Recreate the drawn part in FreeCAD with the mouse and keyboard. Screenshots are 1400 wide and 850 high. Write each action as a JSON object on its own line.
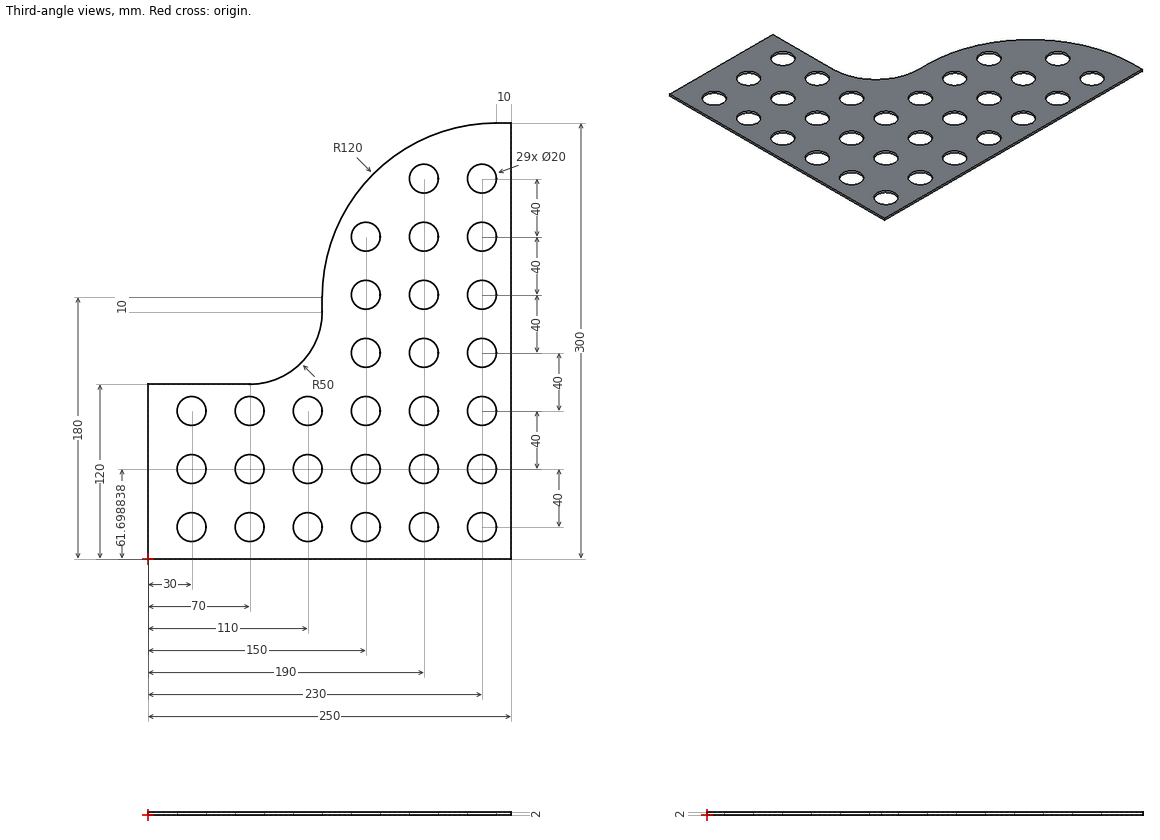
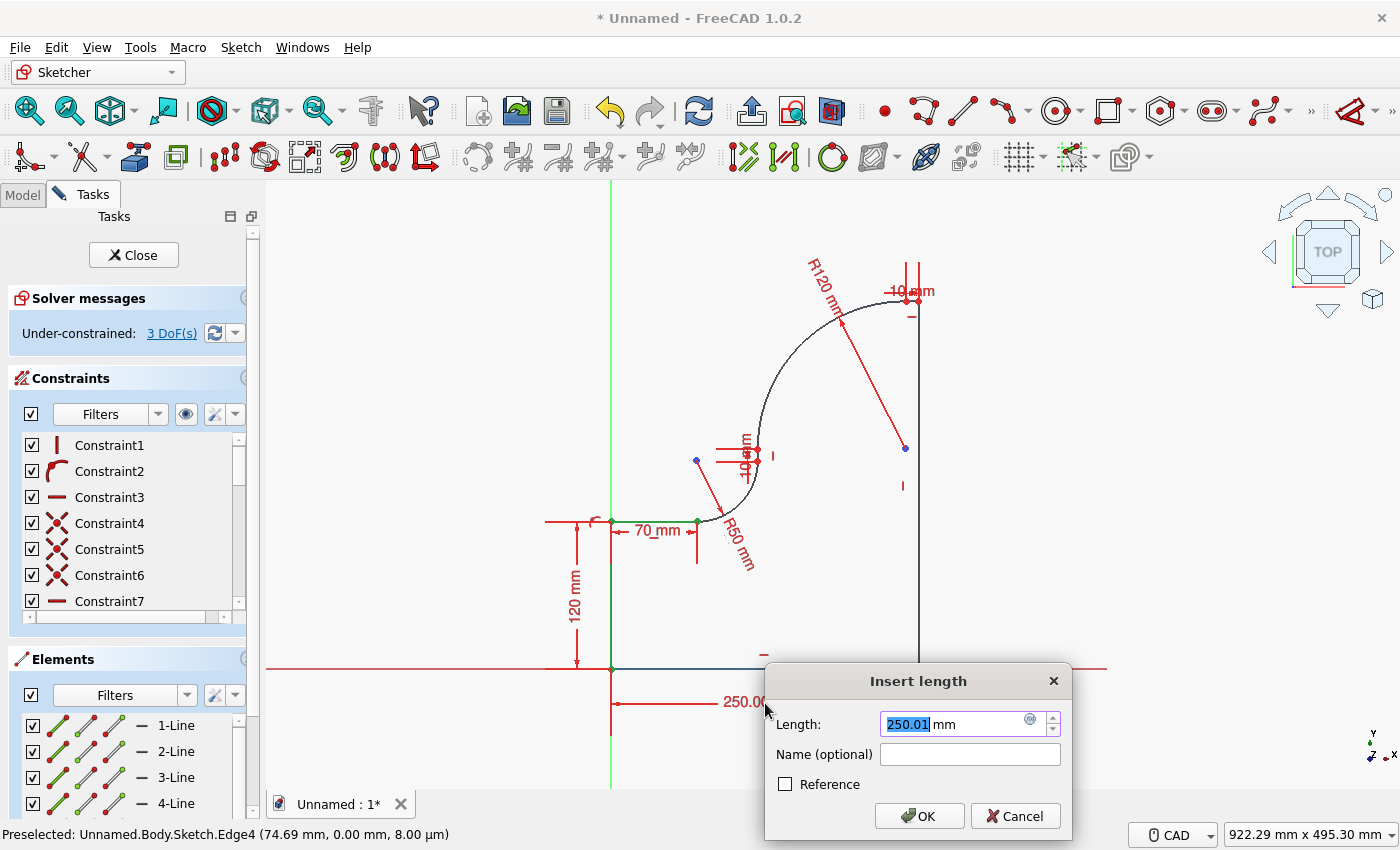
{"action": "type", "text": "250"}
{"action": "key", "text": "Return"}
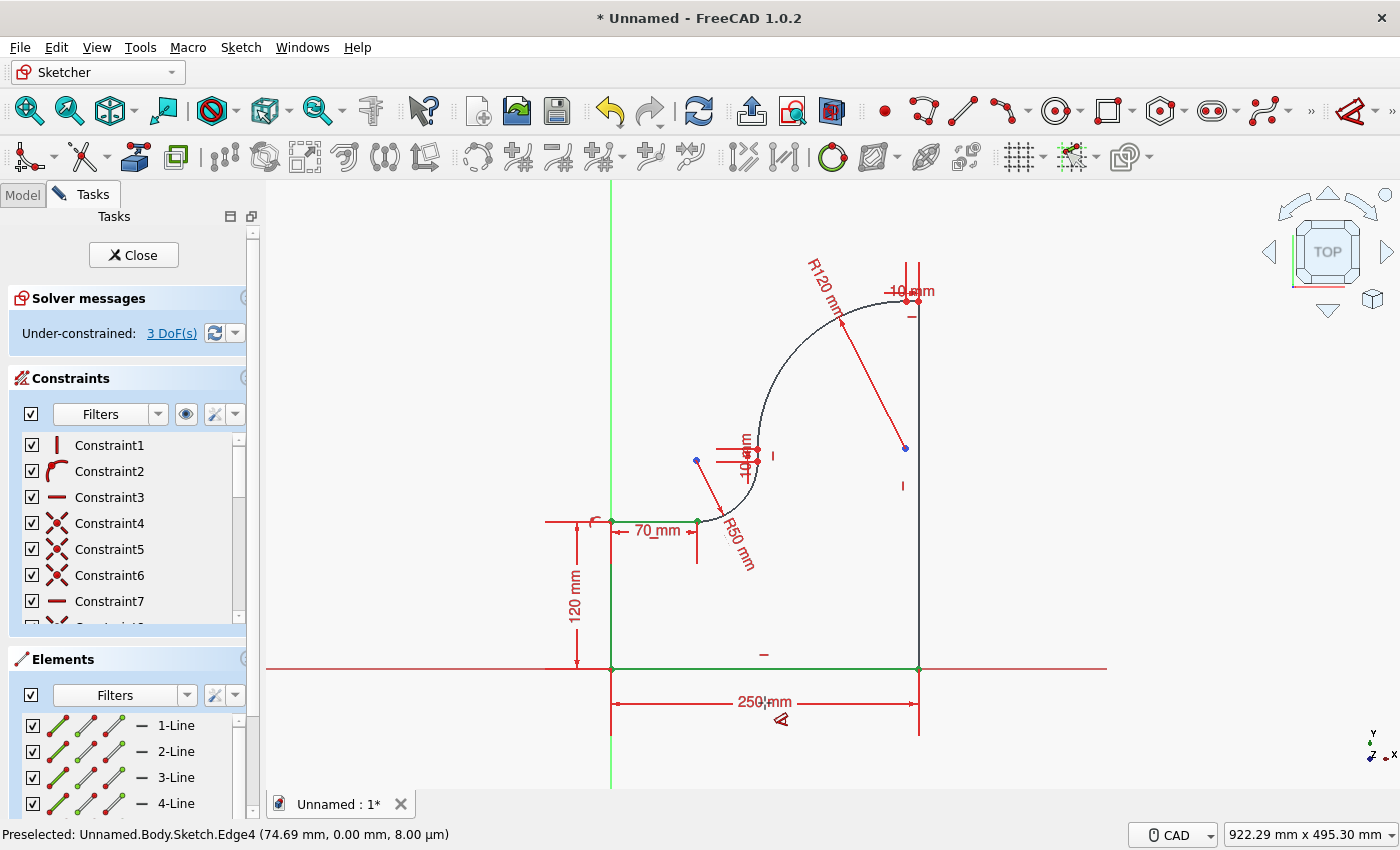
{"action": "left_click", "coordinate": [919, 559]}
{"action": "left_click", "coordinate": [953, 485]}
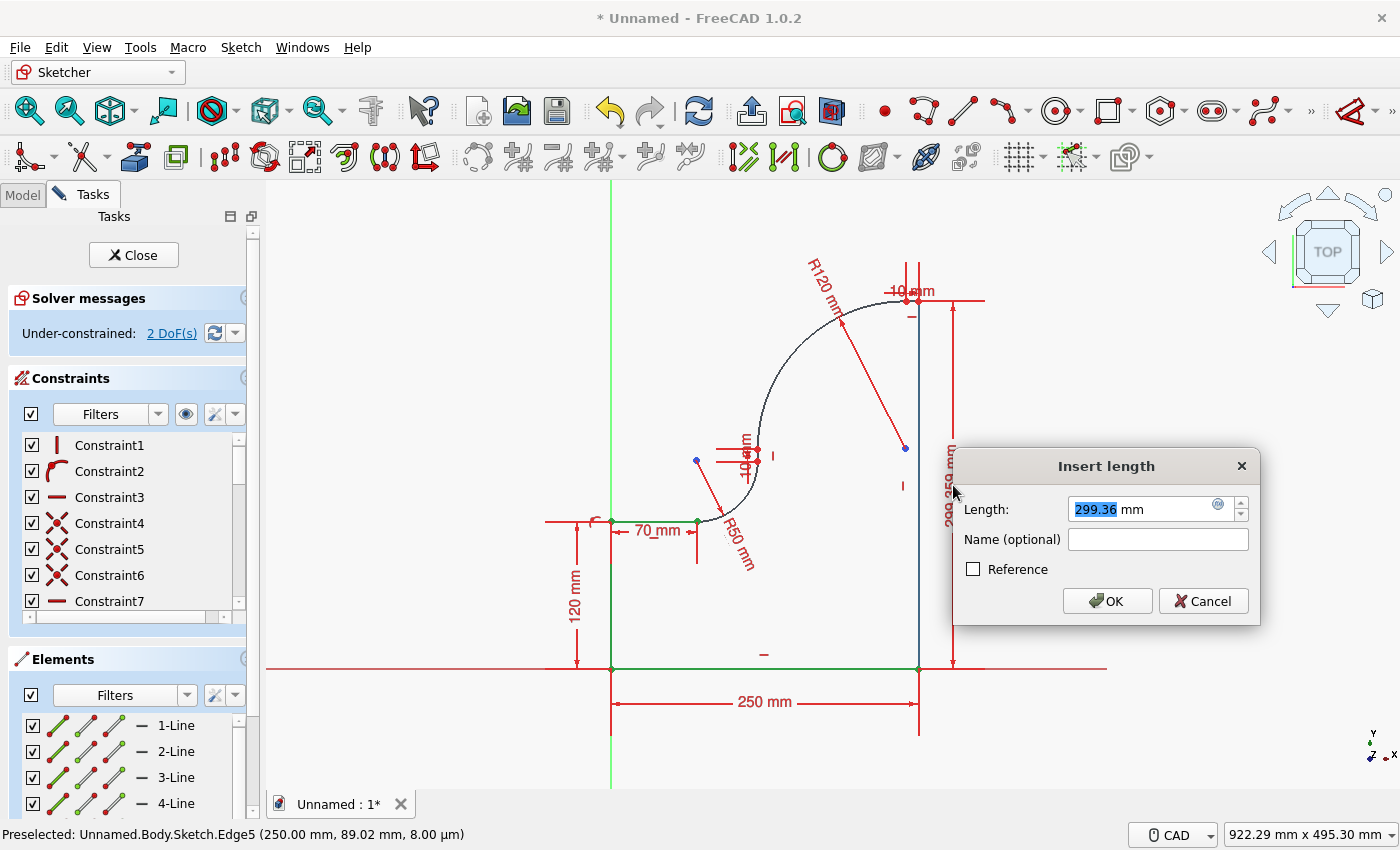
{"action": "type", "text": "300"}
{"action": "key", "text": "Return"}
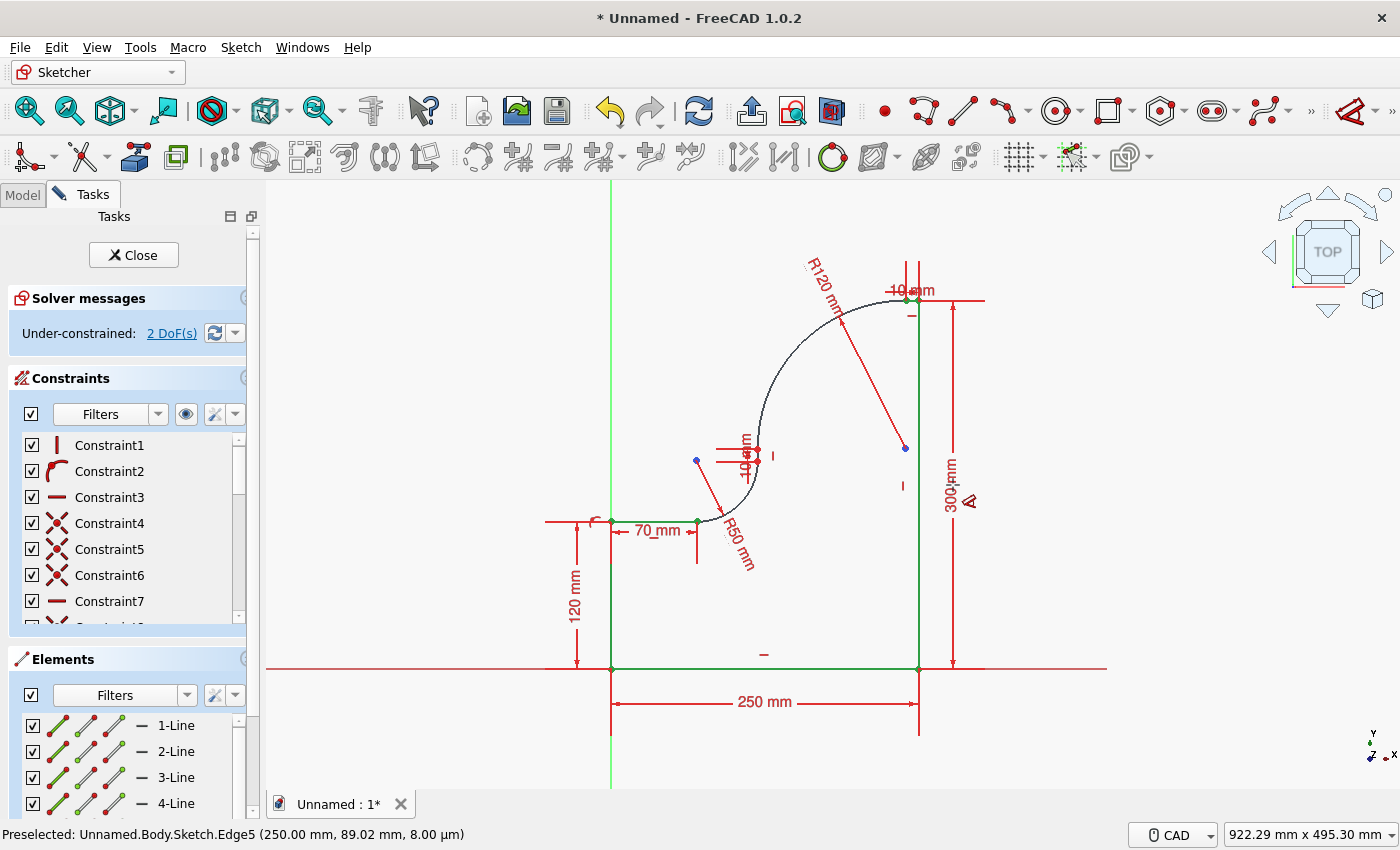
{"action": "left_click", "coordinate": [696, 460]}
{"action": "left_click", "coordinate": [654, 703]}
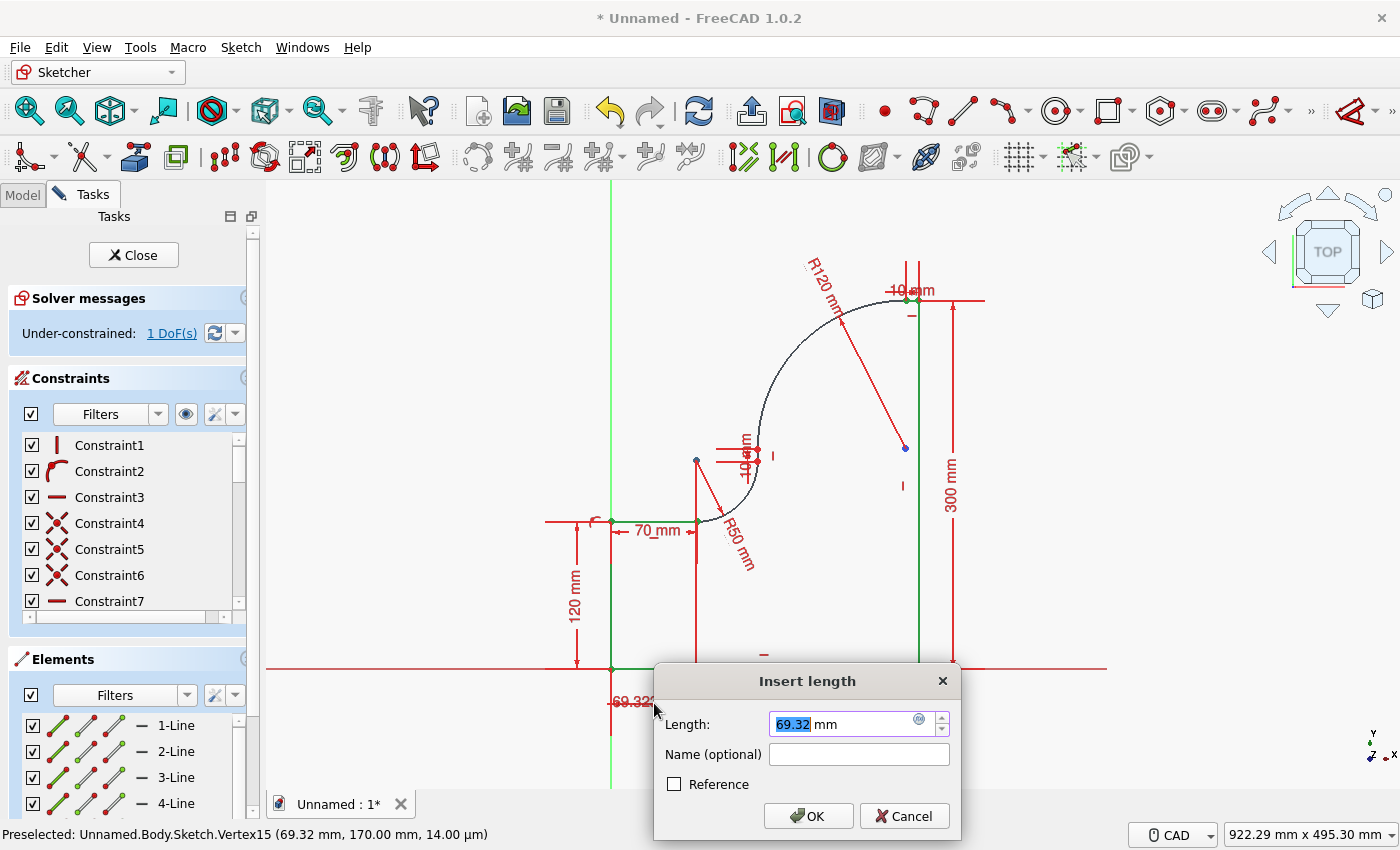
{"action": "type", "text": "70"}
{"action": "key", "text": "Return"}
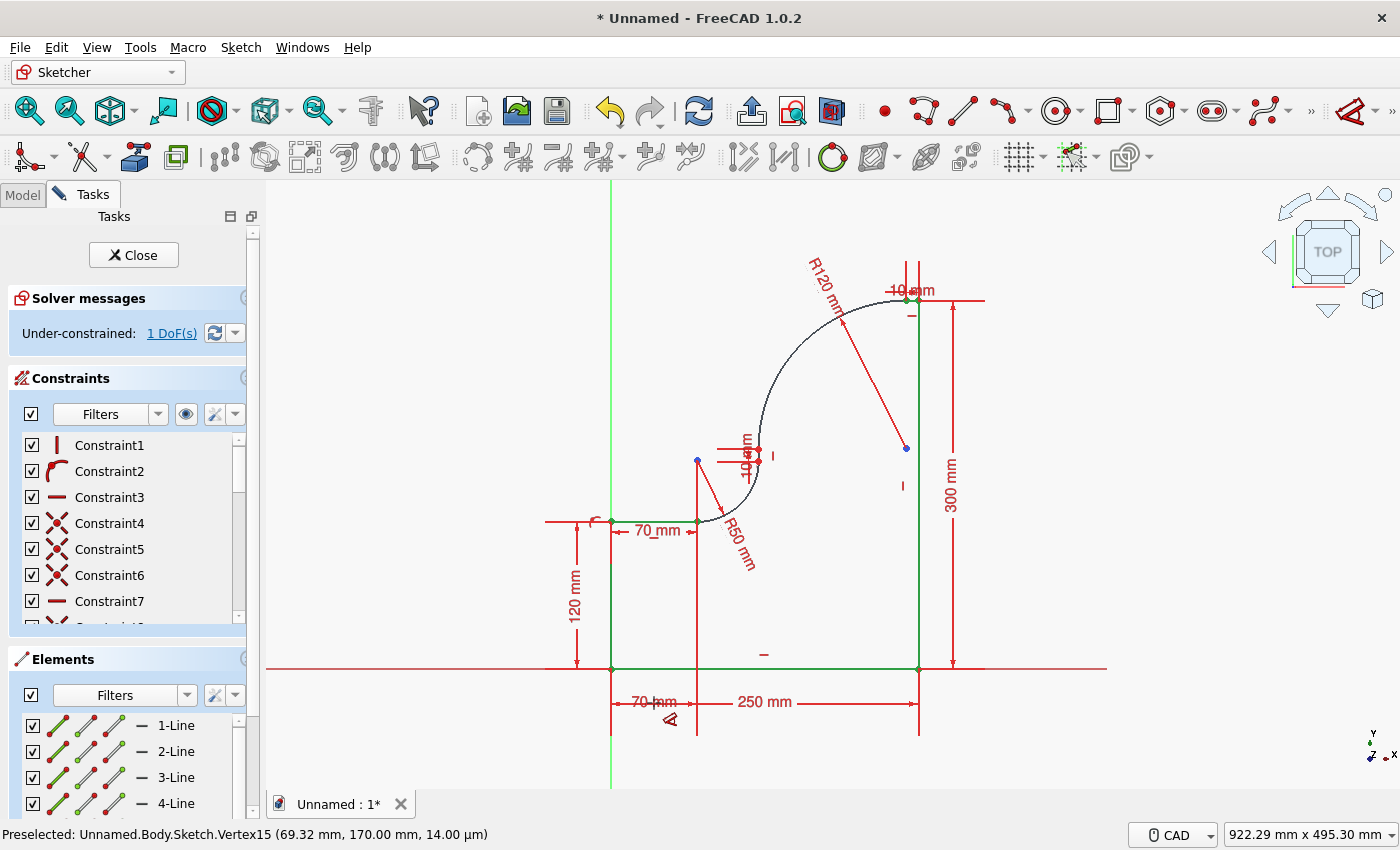
{"action": "left_click", "coordinate": [759, 449]}
{"action": "left_click", "coordinate": [577, 559]}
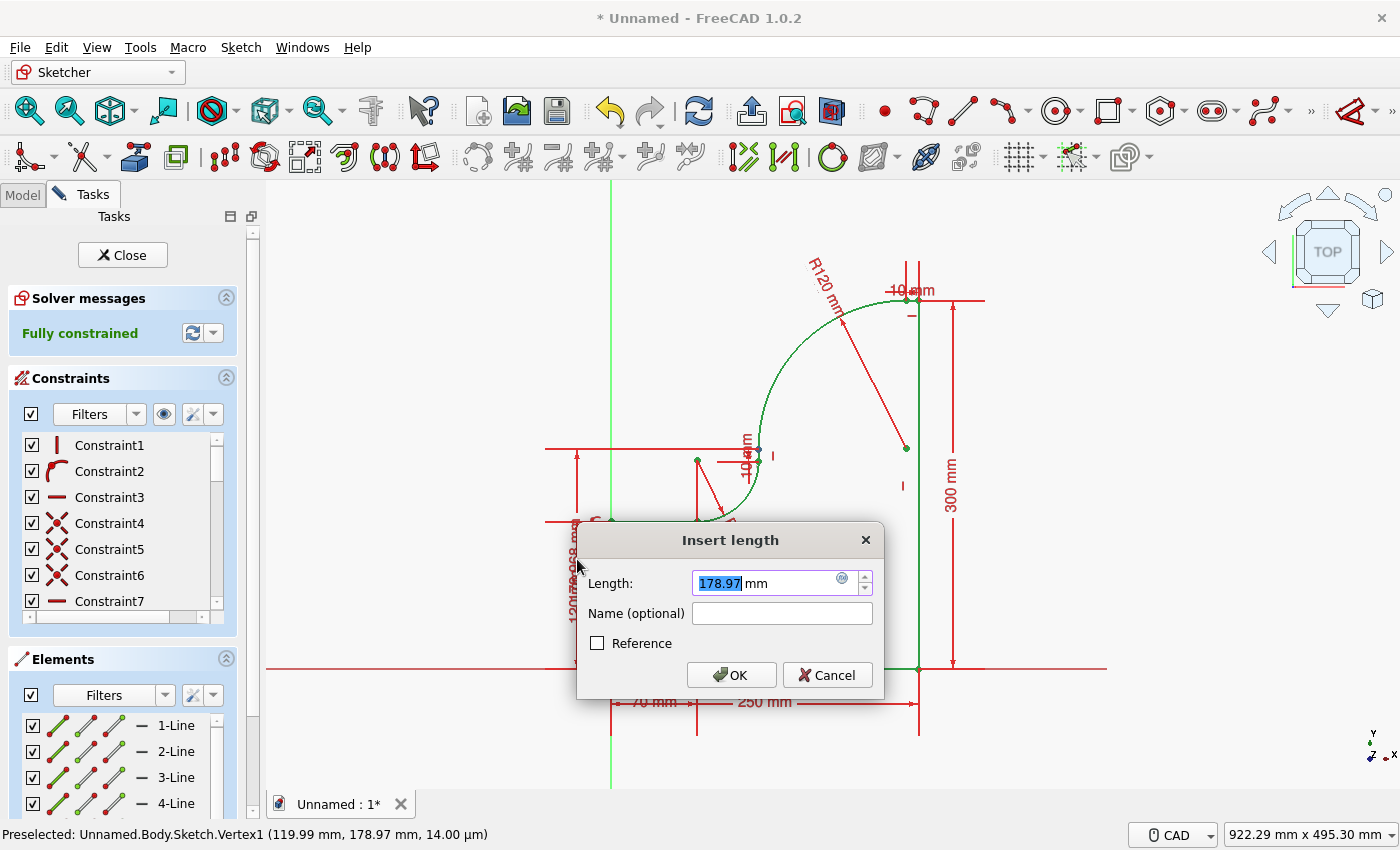
{"action": "type", "text": "180"}
{"action": "key", "text": "Return"}
{"action": "key", "text": "Escape"}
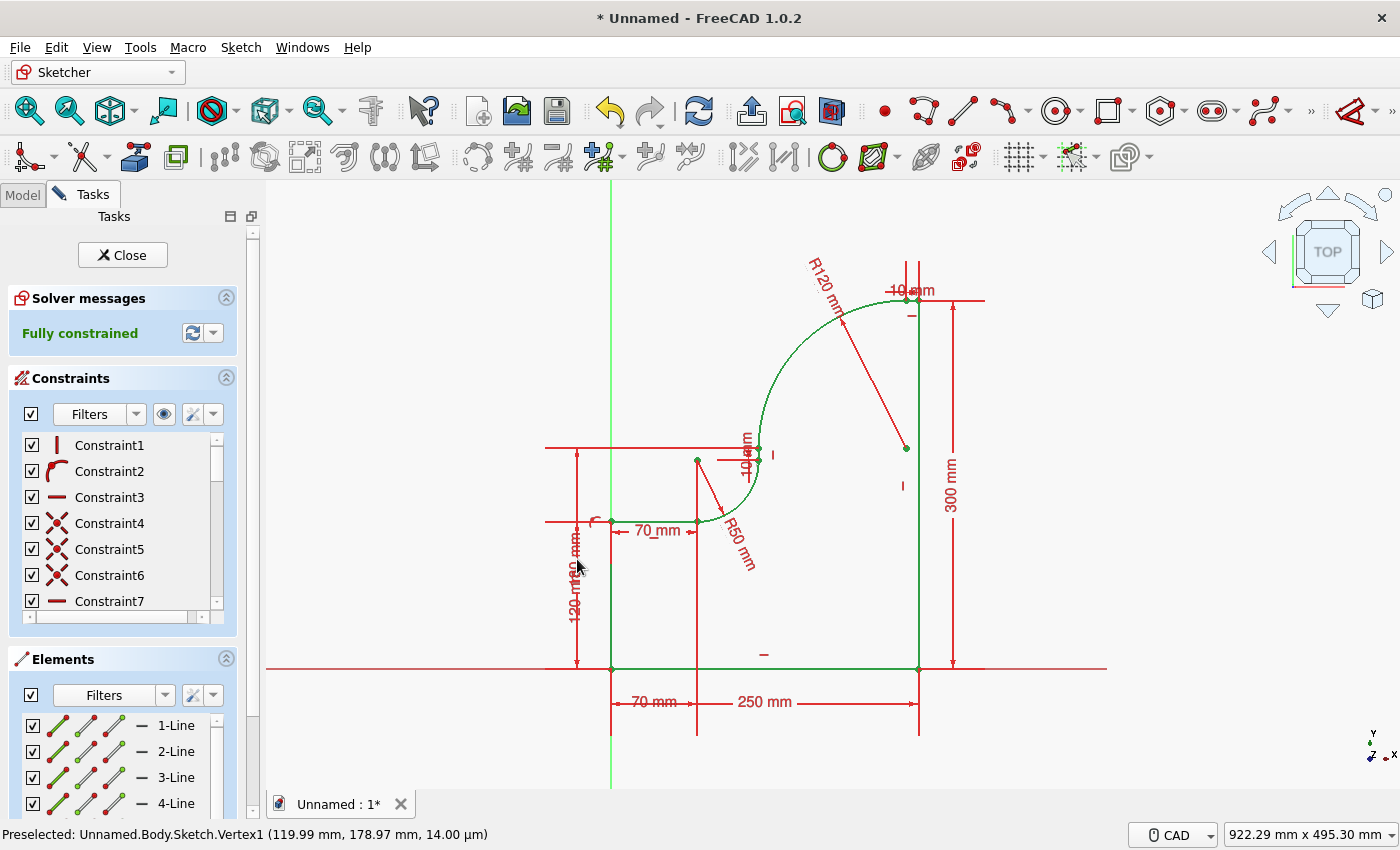
{"action": "left_click", "coordinate": [123, 255]}